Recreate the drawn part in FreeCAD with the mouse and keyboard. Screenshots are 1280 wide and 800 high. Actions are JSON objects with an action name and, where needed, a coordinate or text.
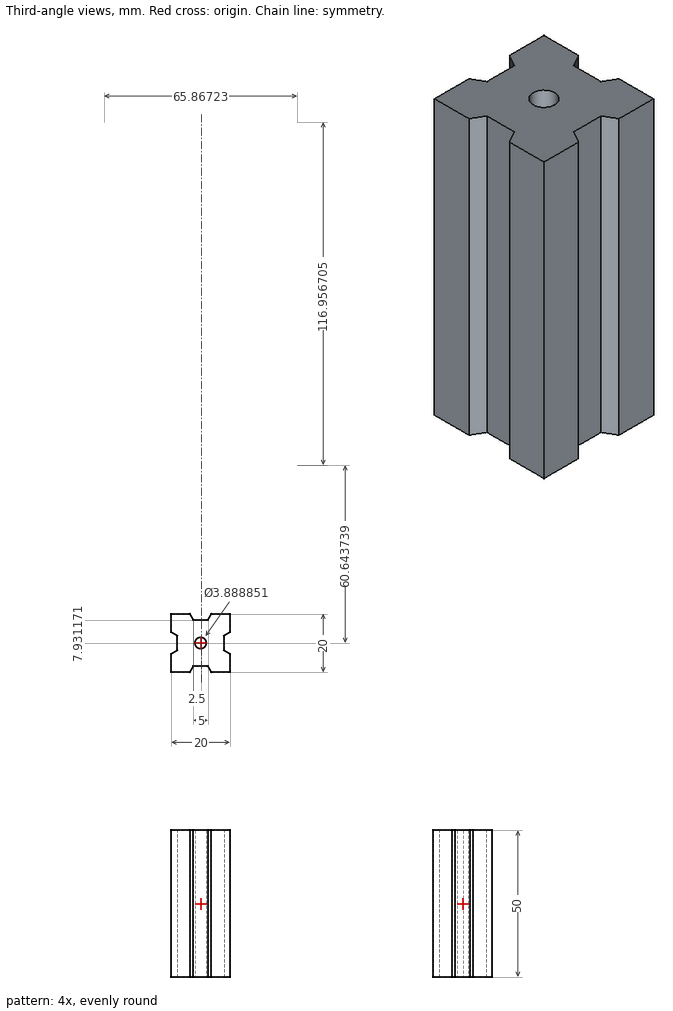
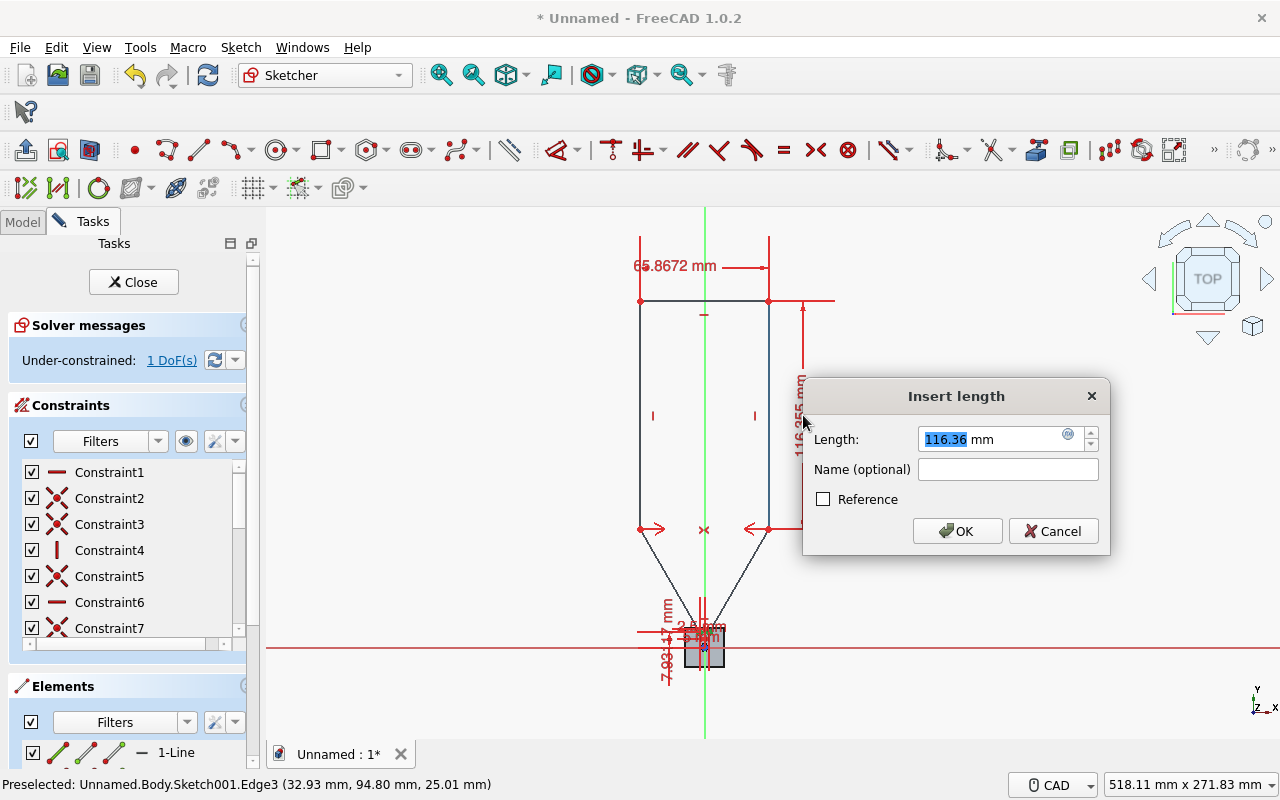
{"action": "type", "text": "116.956705"}
{"action": "key", "text": "Return"}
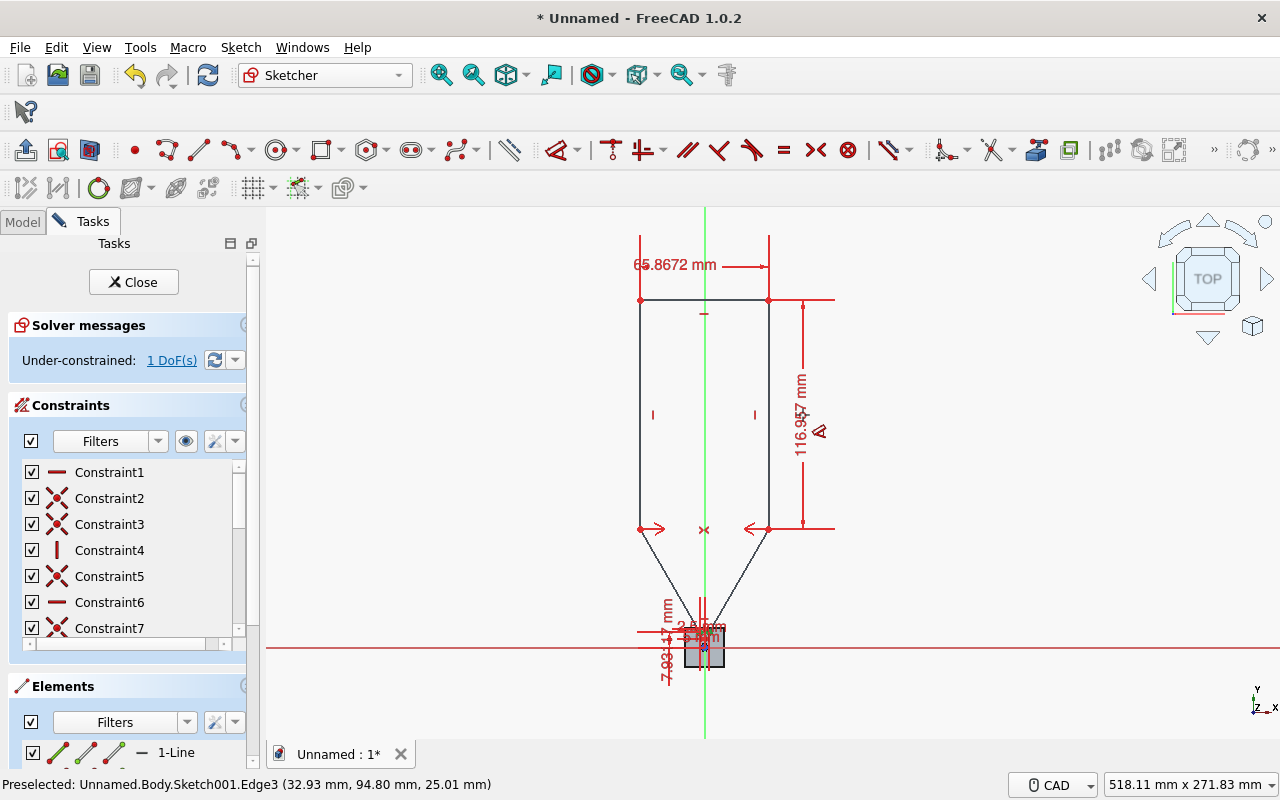
{"action": "left_click", "coordinate": [769, 529]}
{"action": "left_click", "coordinate": [803, 588]}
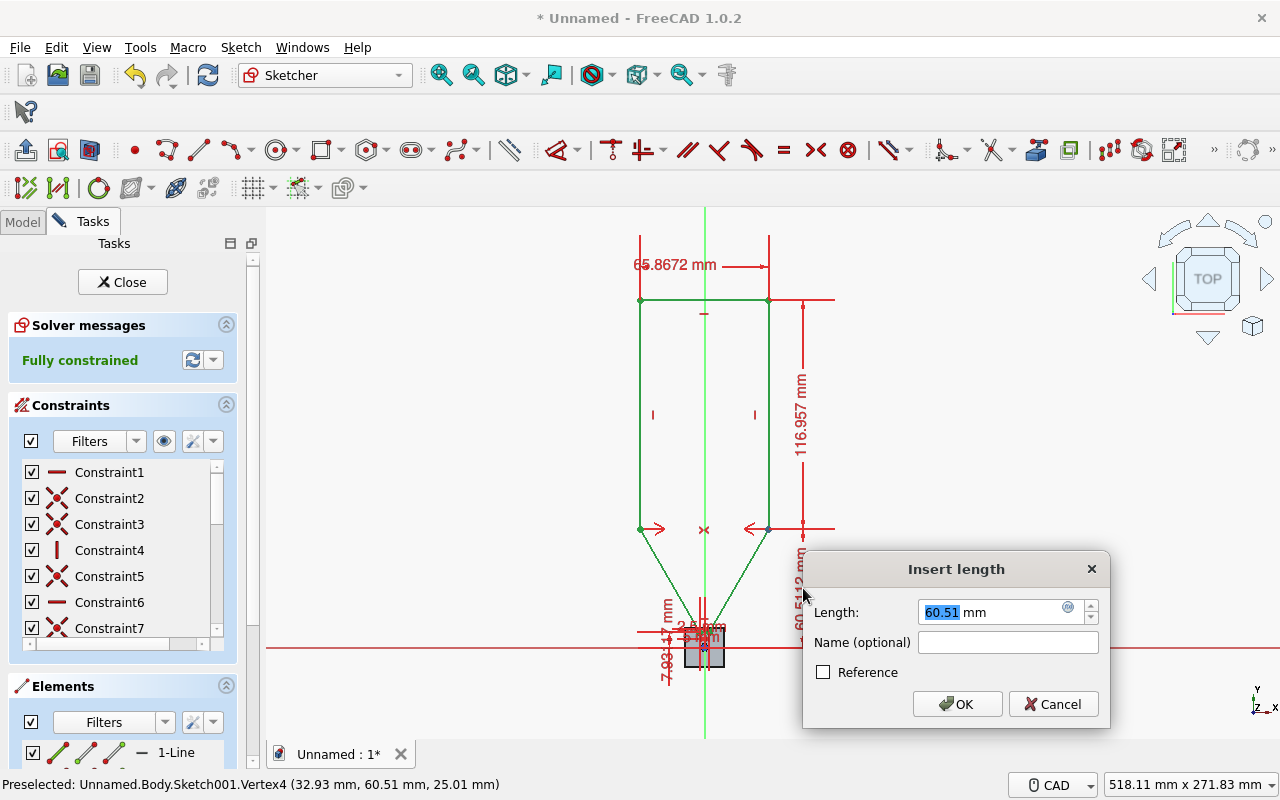
{"action": "type", "text": "60.643739"}
{"action": "key", "text": "Return"}
{"action": "key", "text": "Escape"}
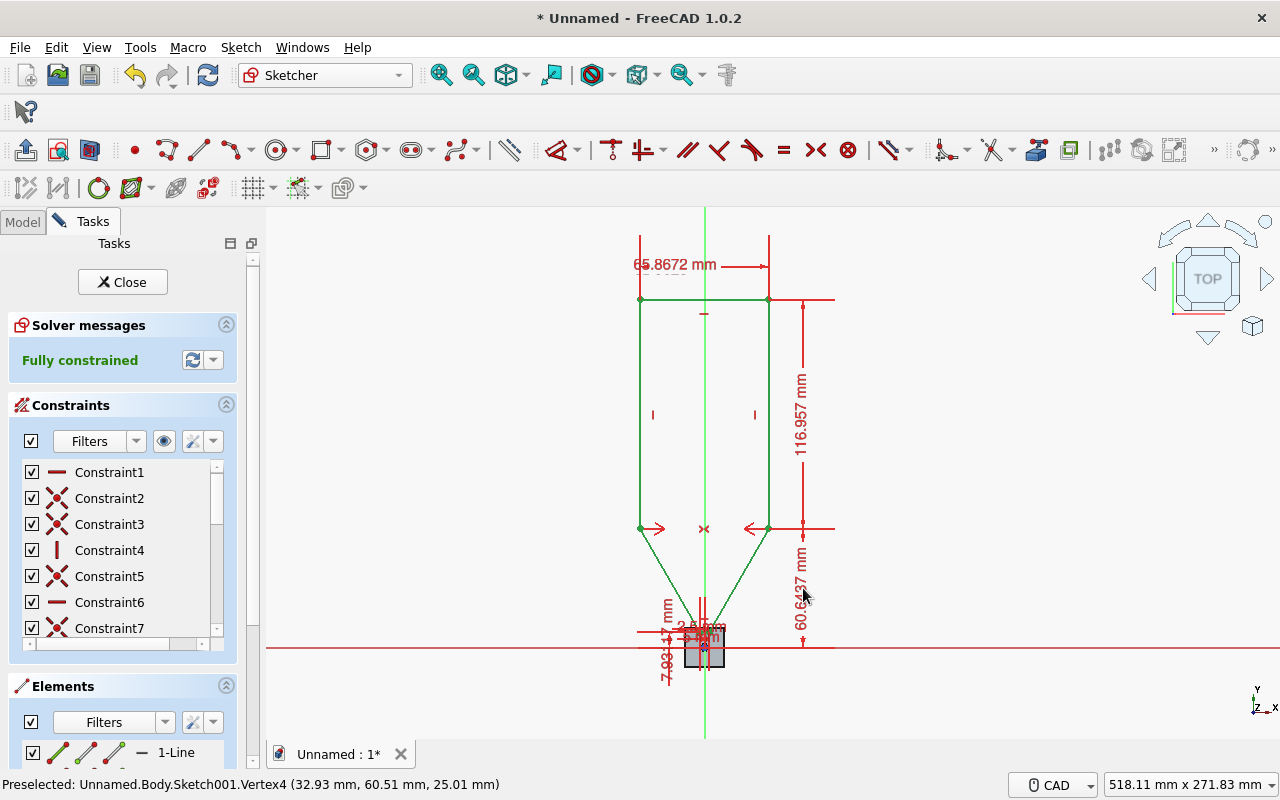
{"action": "left_click", "coordinate": [123, 282]}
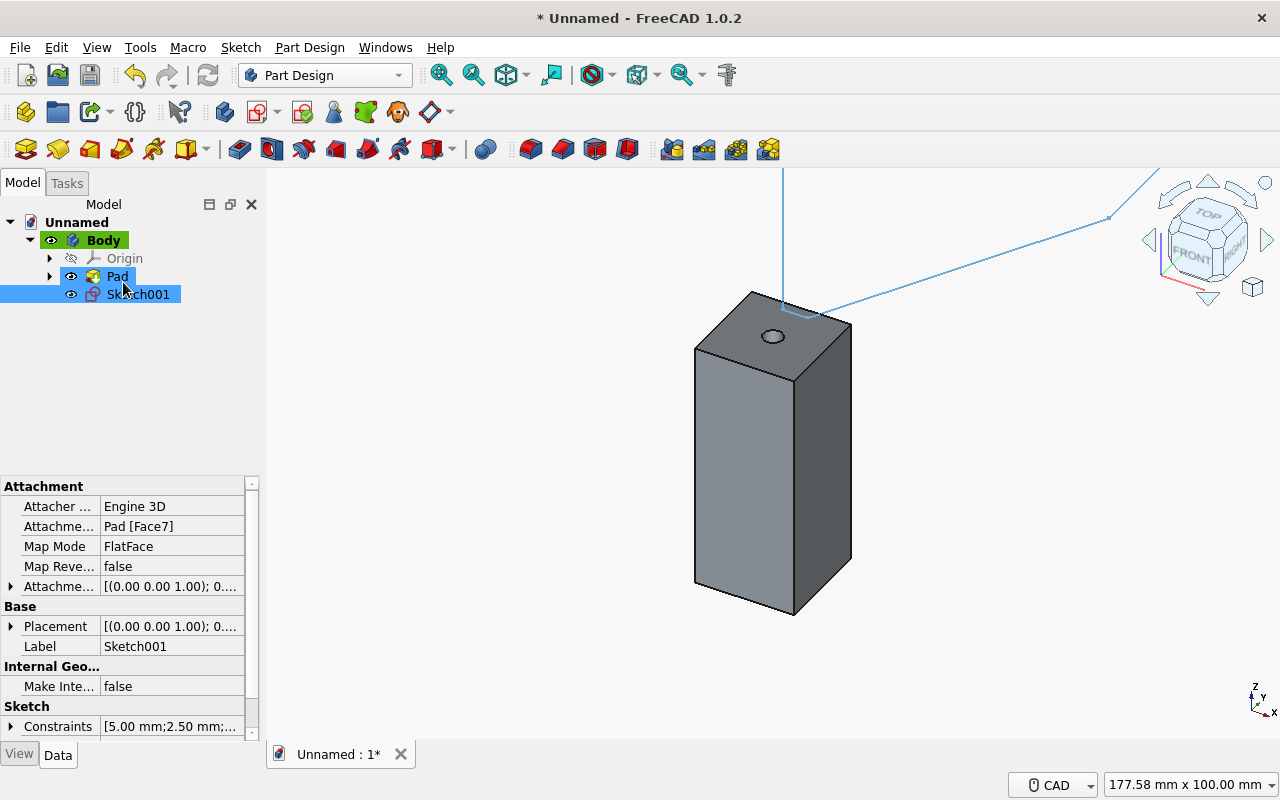
{"action": "left_click", "coordinate": [240, 150]}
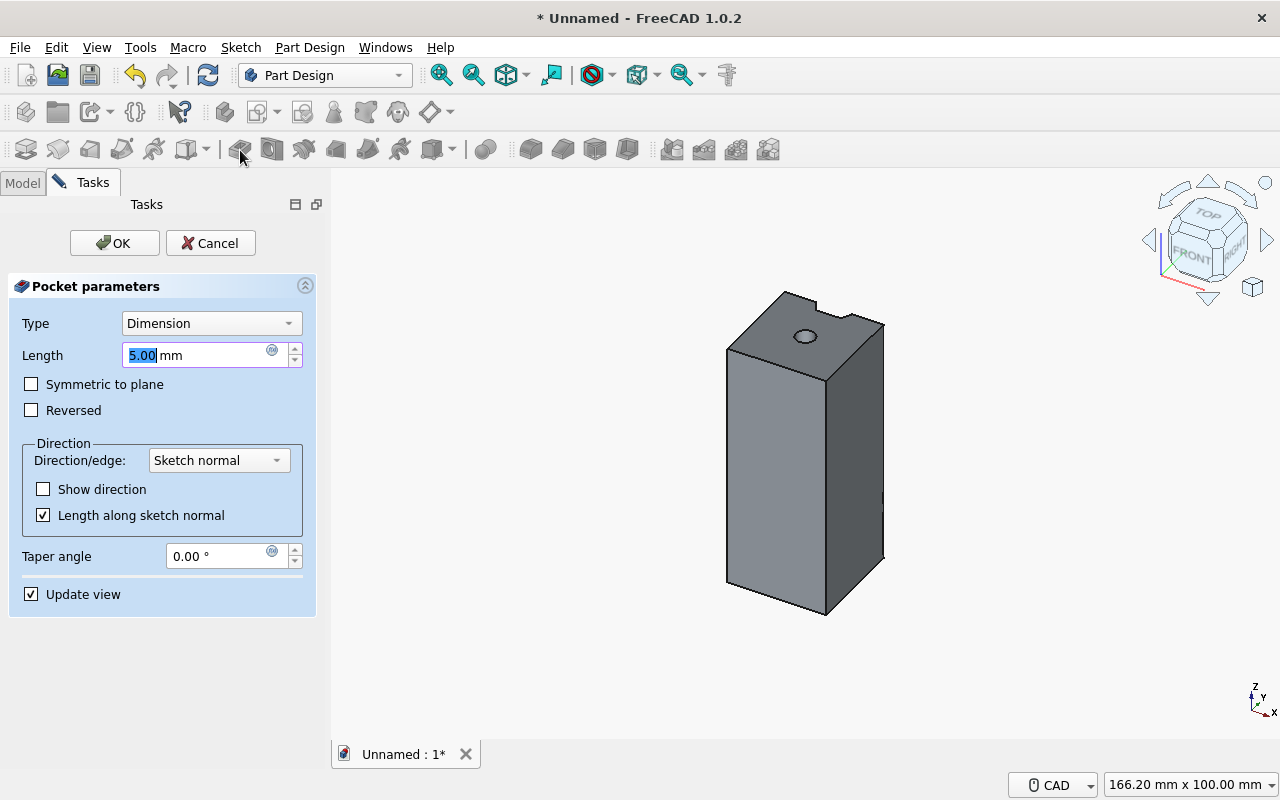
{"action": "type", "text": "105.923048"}
{"action": "key", "text": "Tab"}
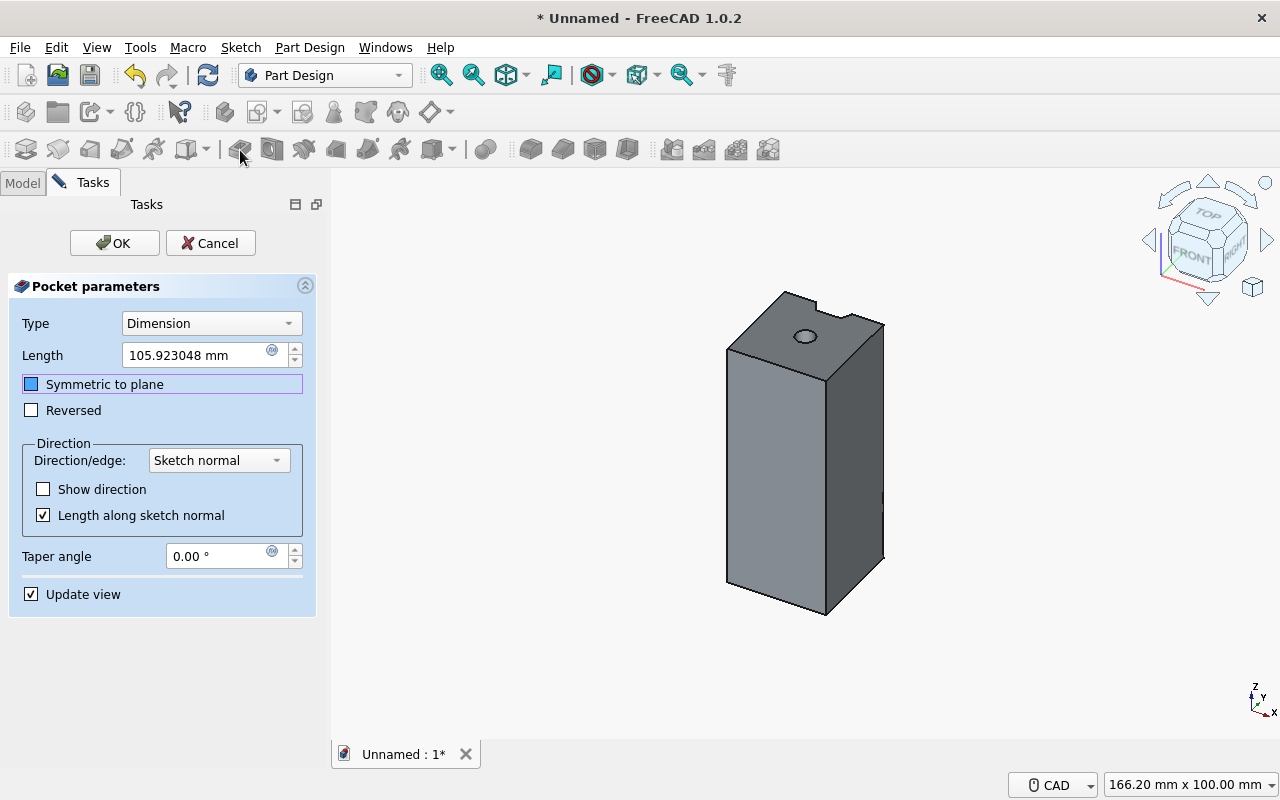
{"action": "left_click", "coordinate": [30, 384]}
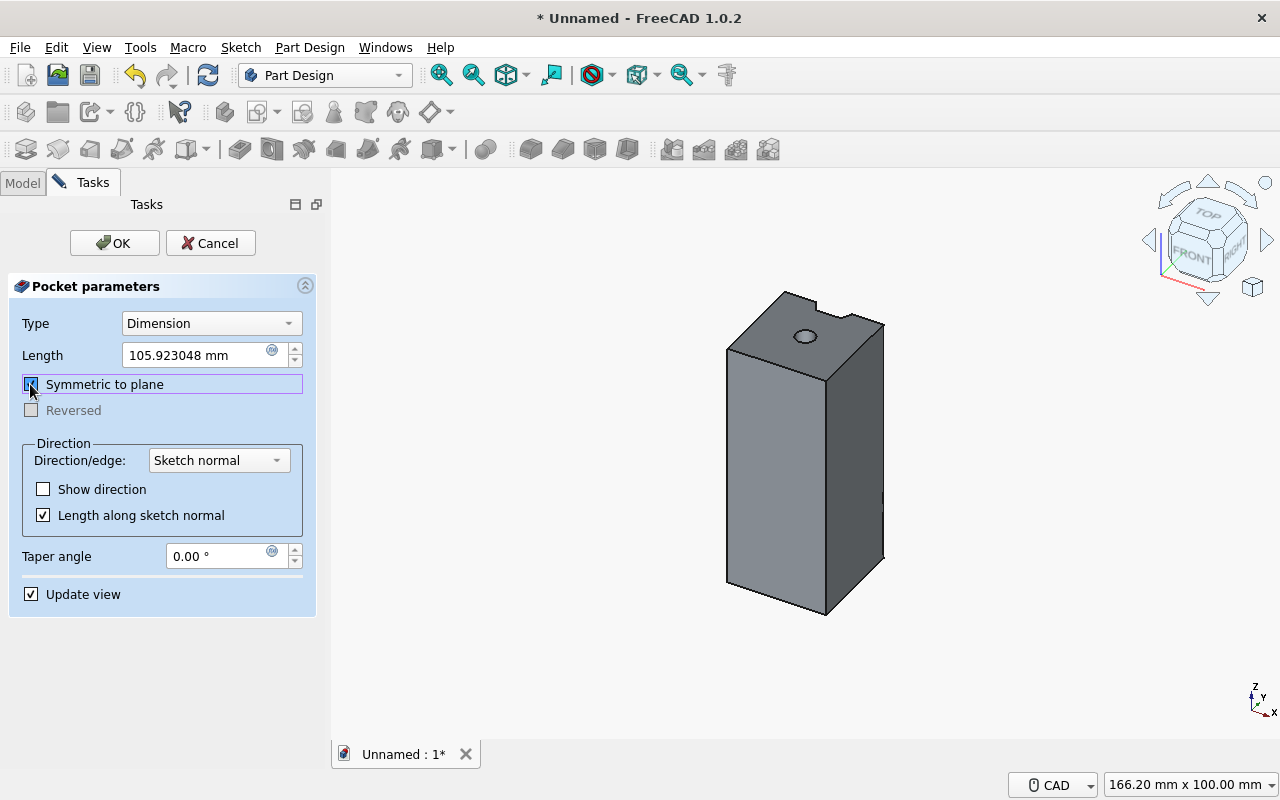
{"action": "left_click", "coordinate": [115, 243]}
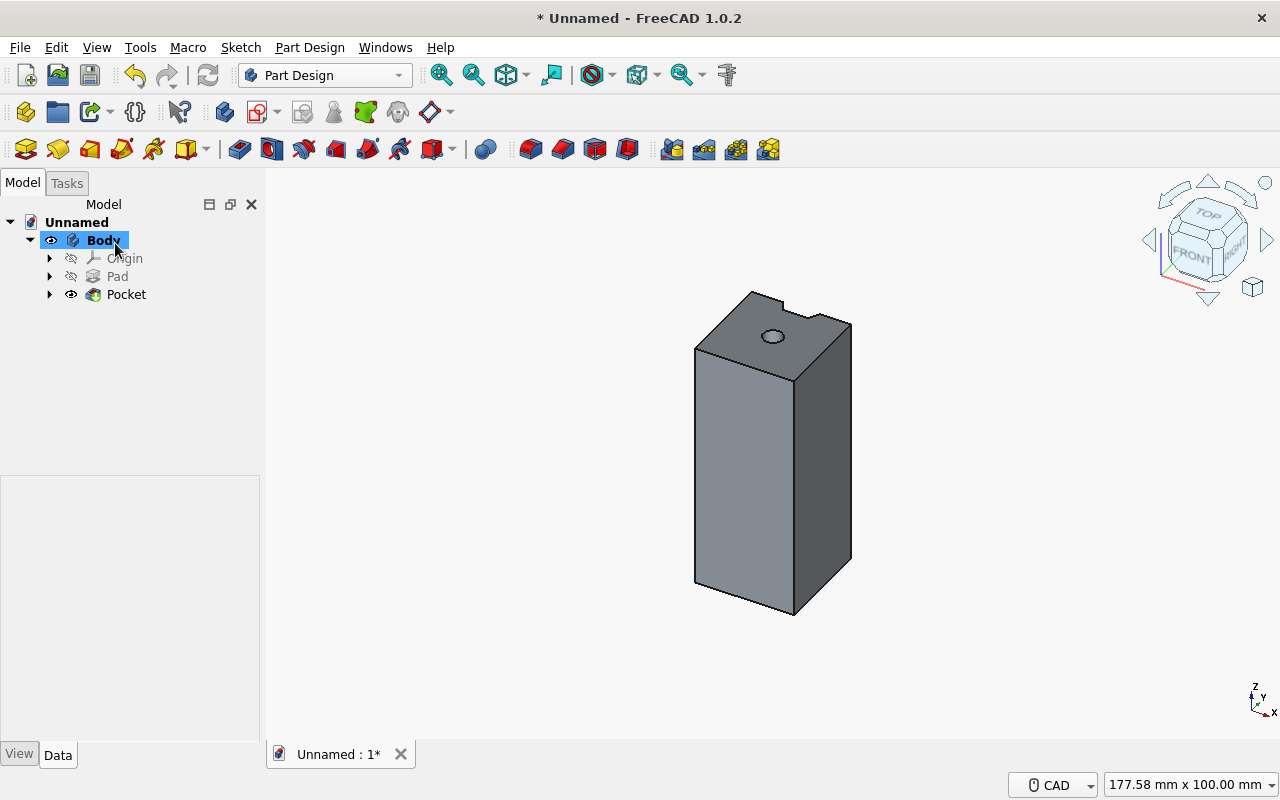
{"action": "left_click", "coordinate": [116, 294]}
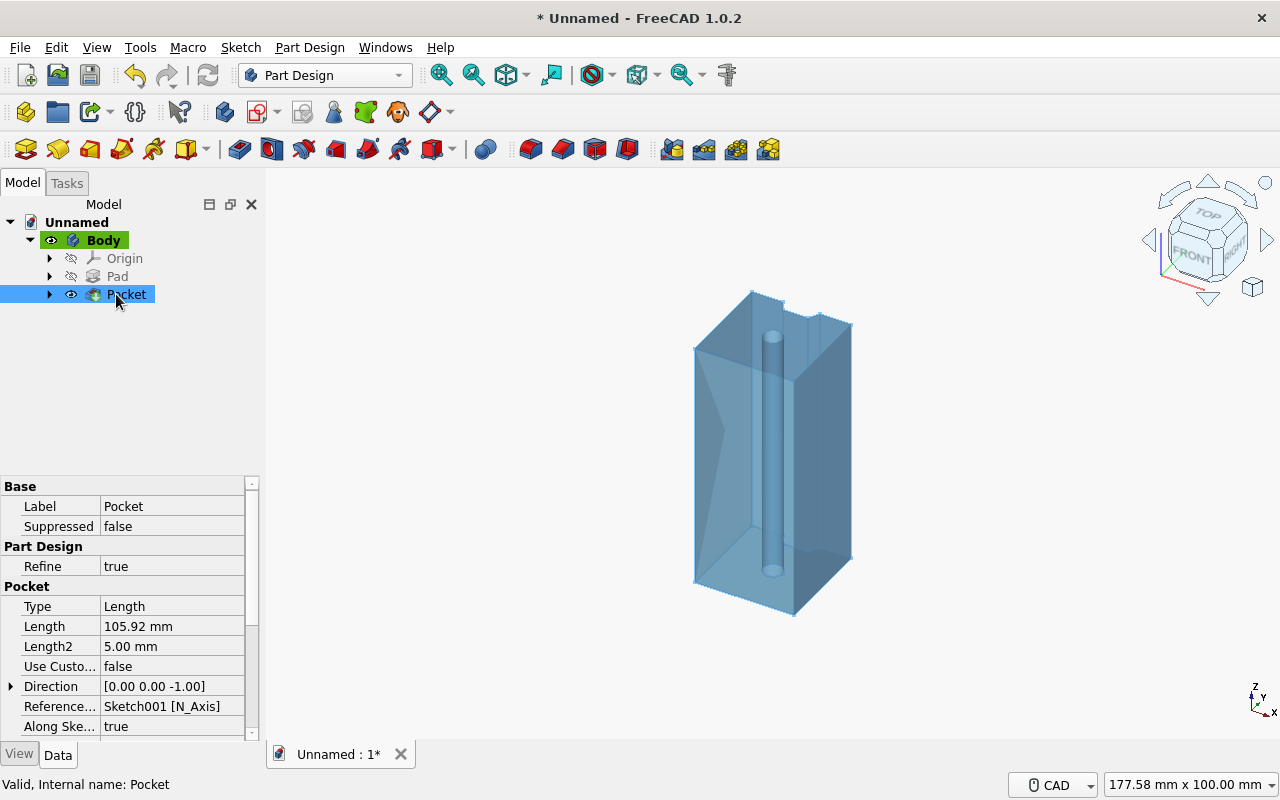
{"action": "left_click", "coordinate": [736, 150]}